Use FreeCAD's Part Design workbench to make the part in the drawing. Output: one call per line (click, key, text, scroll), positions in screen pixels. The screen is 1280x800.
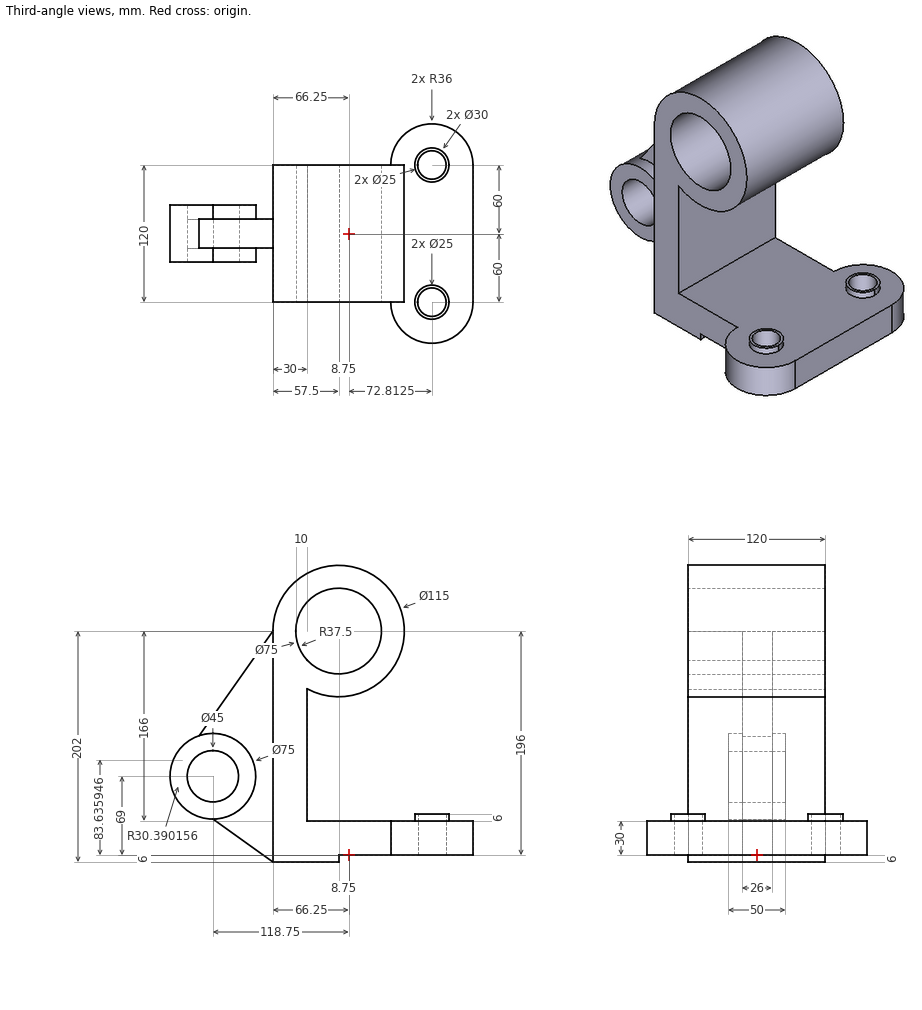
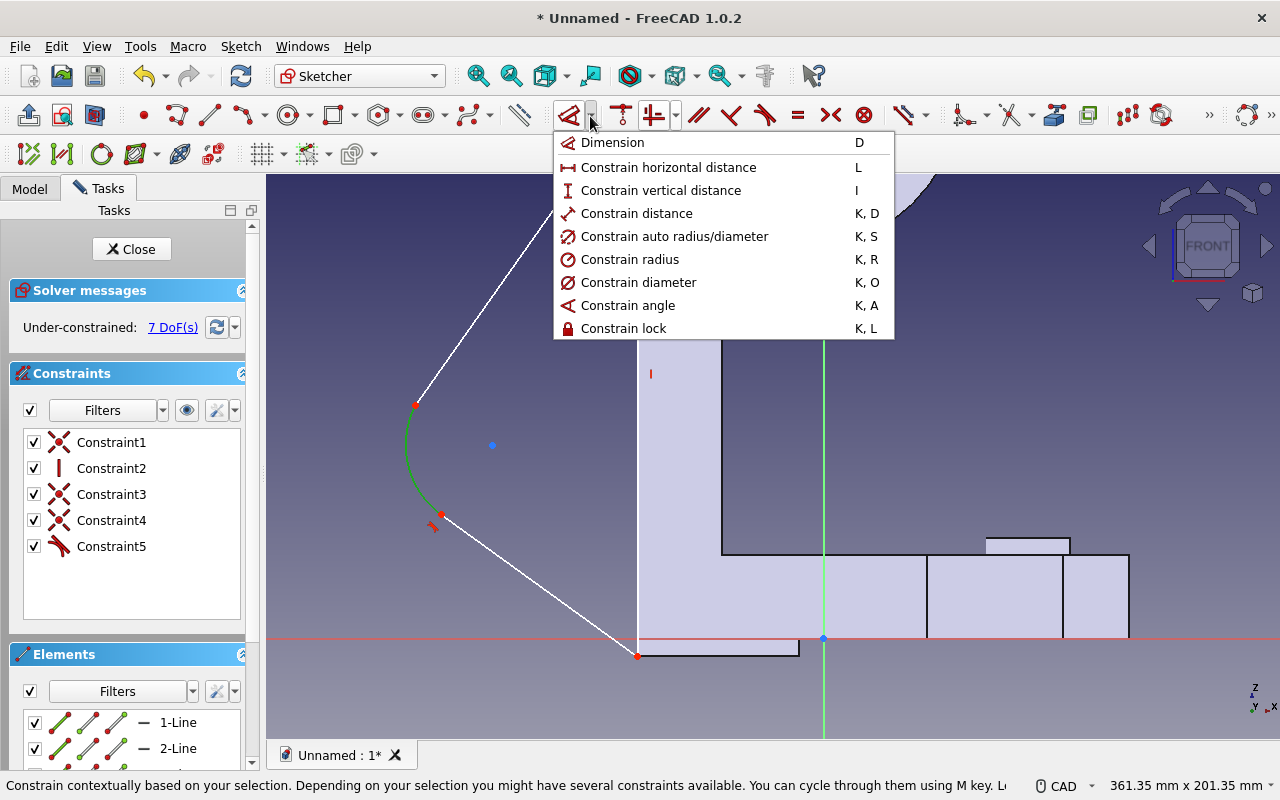
click(724, 260)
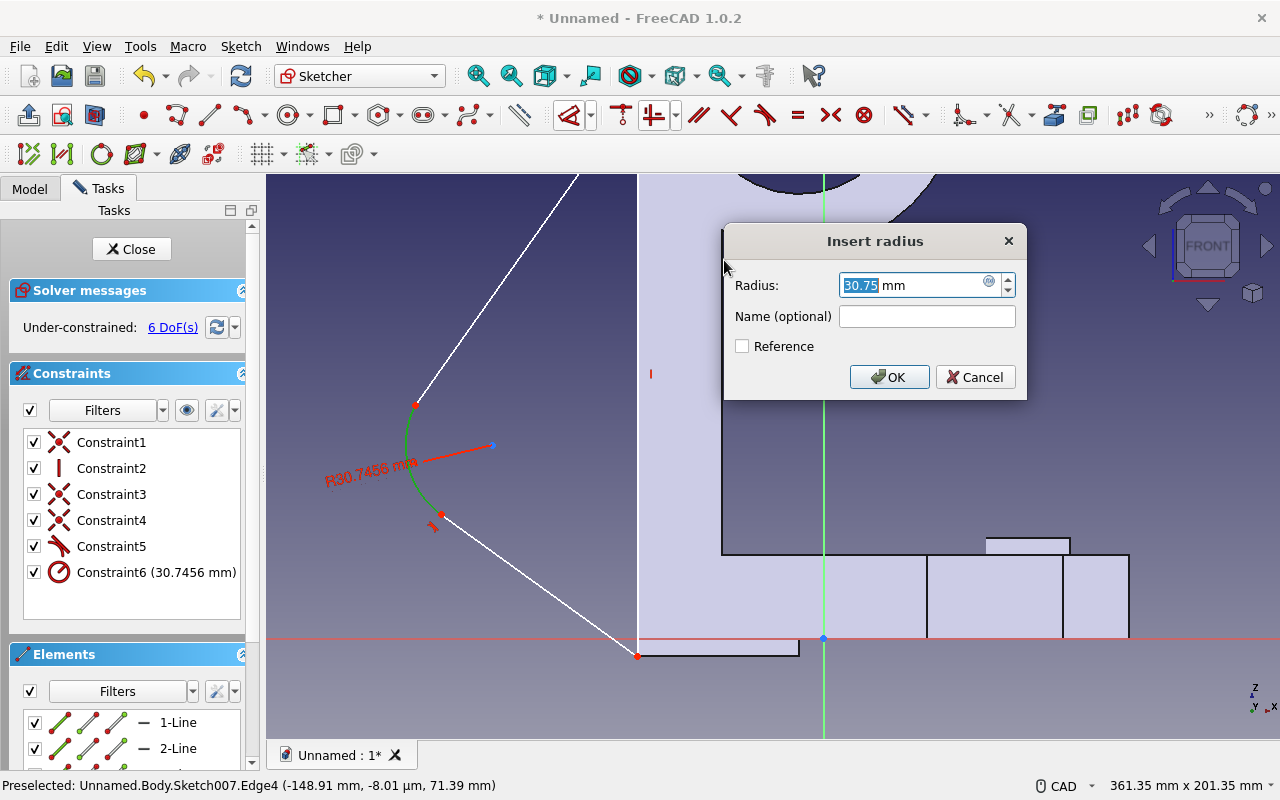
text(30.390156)
key(Return)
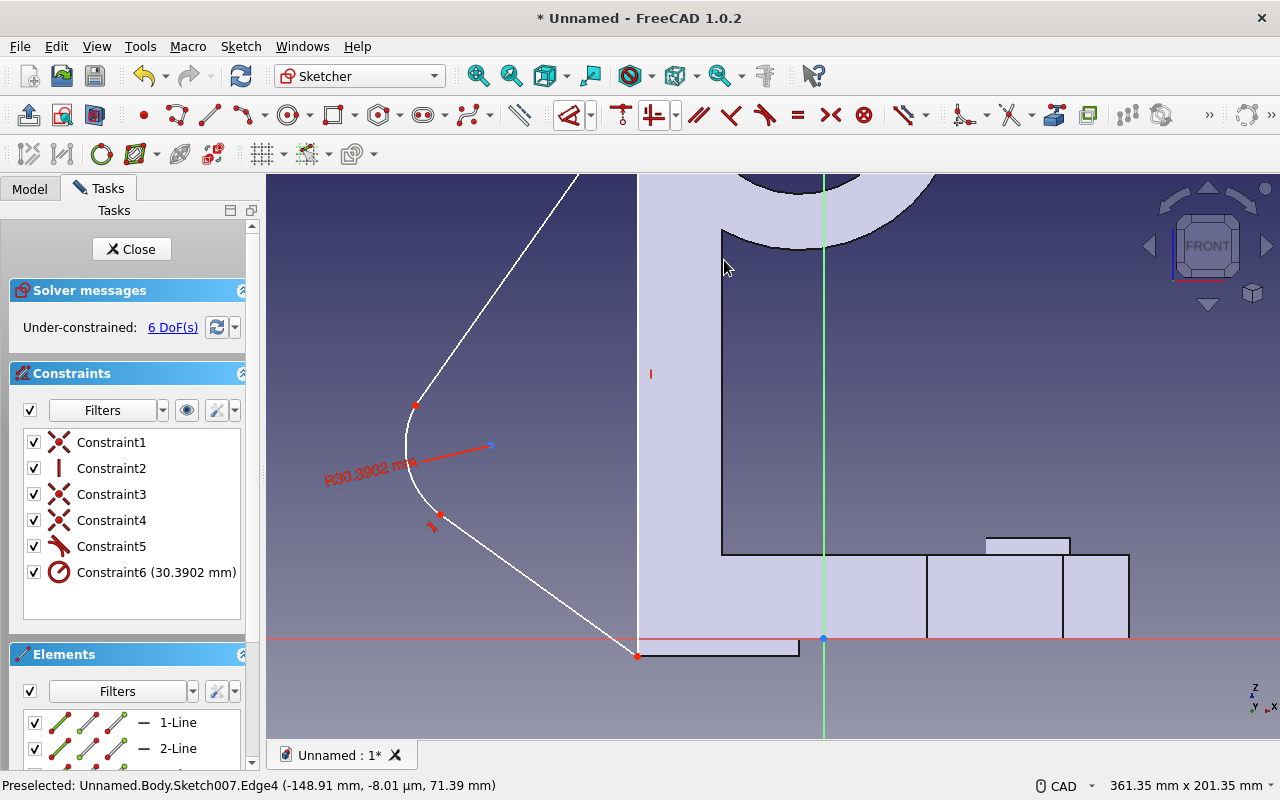
scroll(638, 657, up, 5)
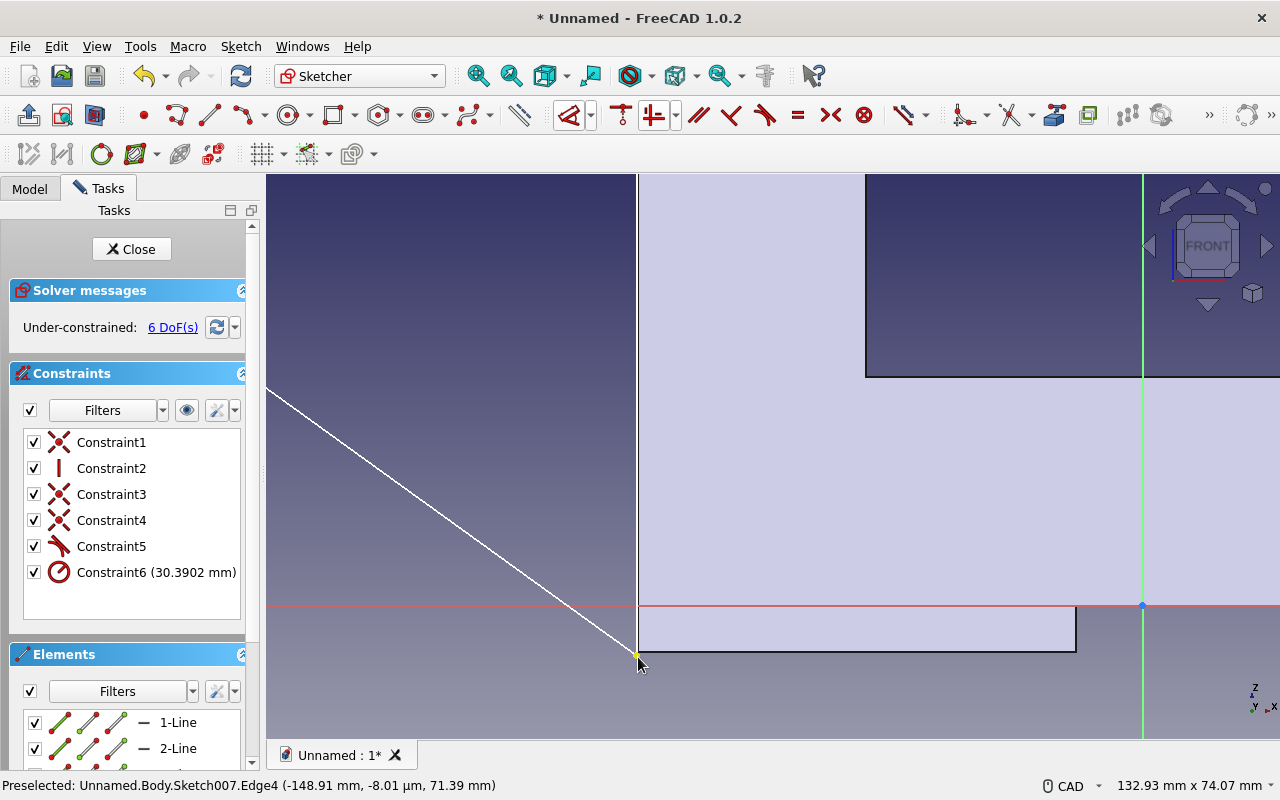
click(637, 656)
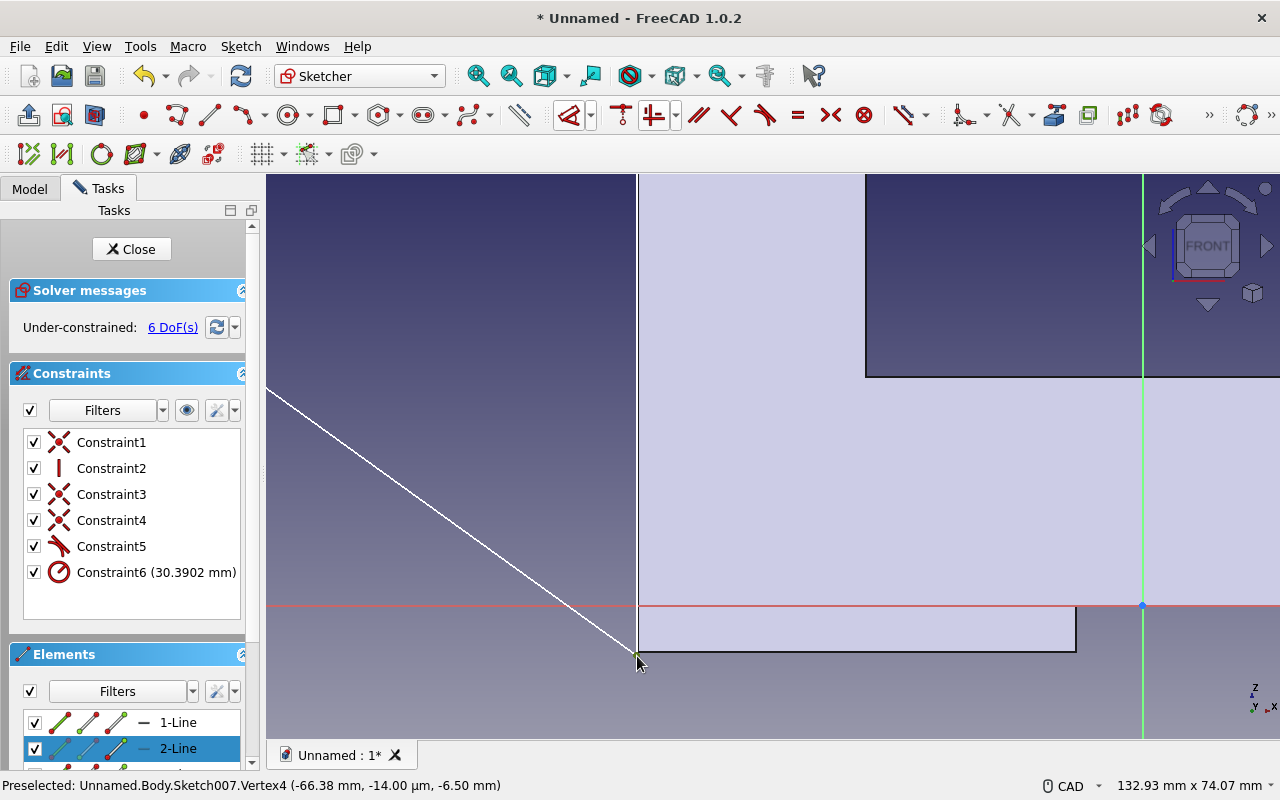
key(i)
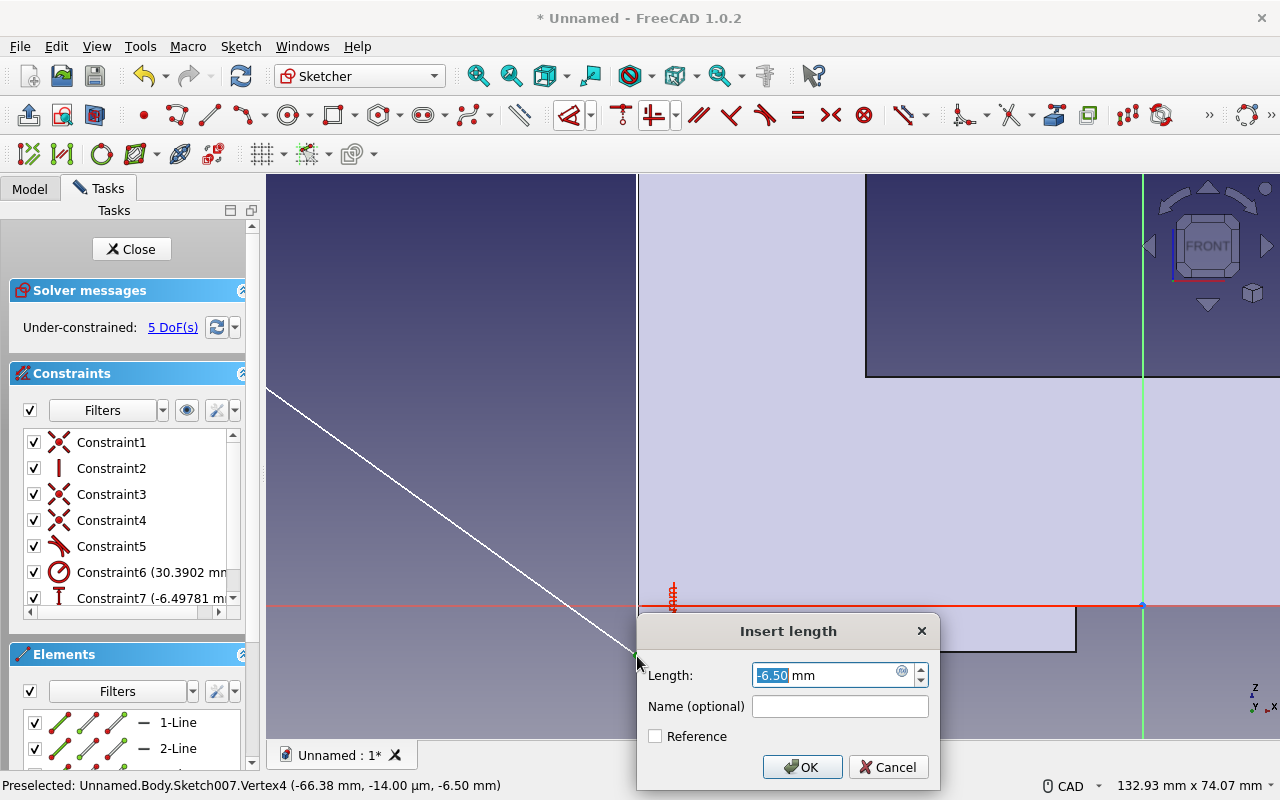
text(-6)
key(Return)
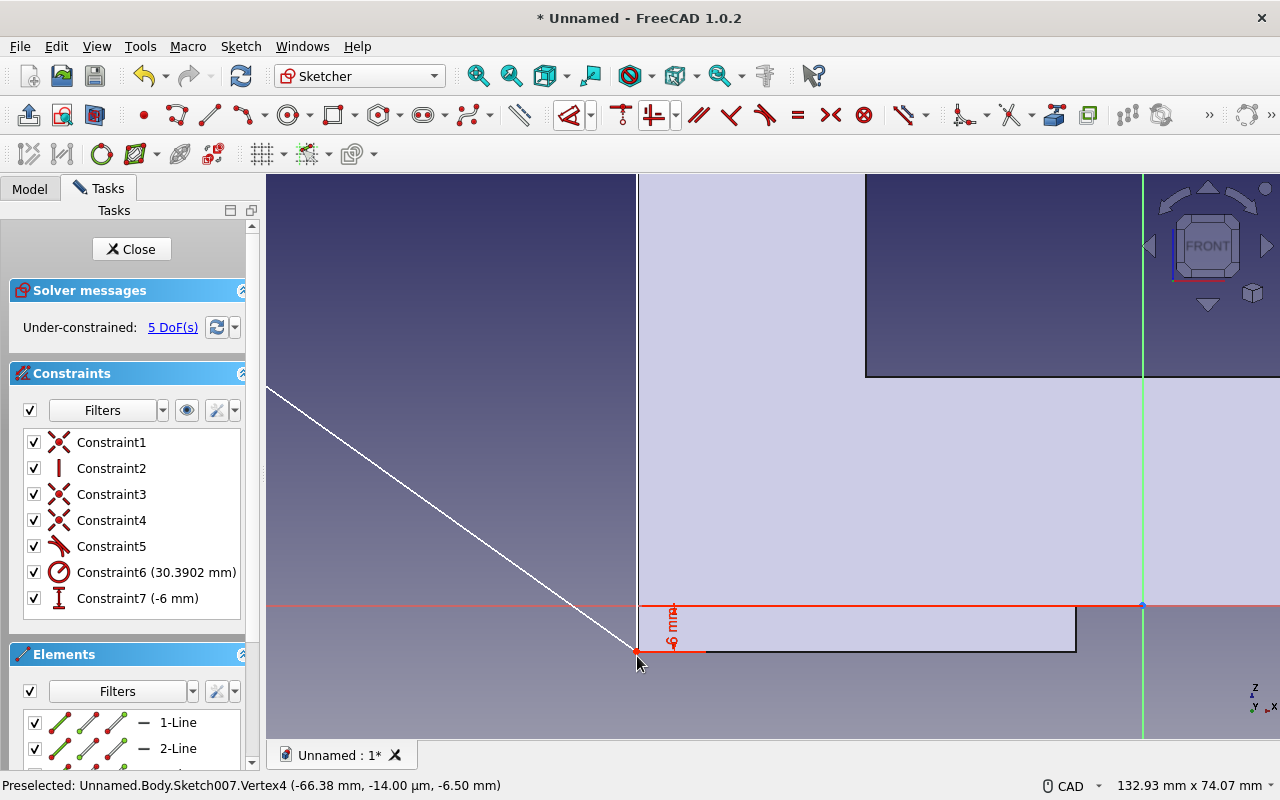
scroll(746, 645, down, 7)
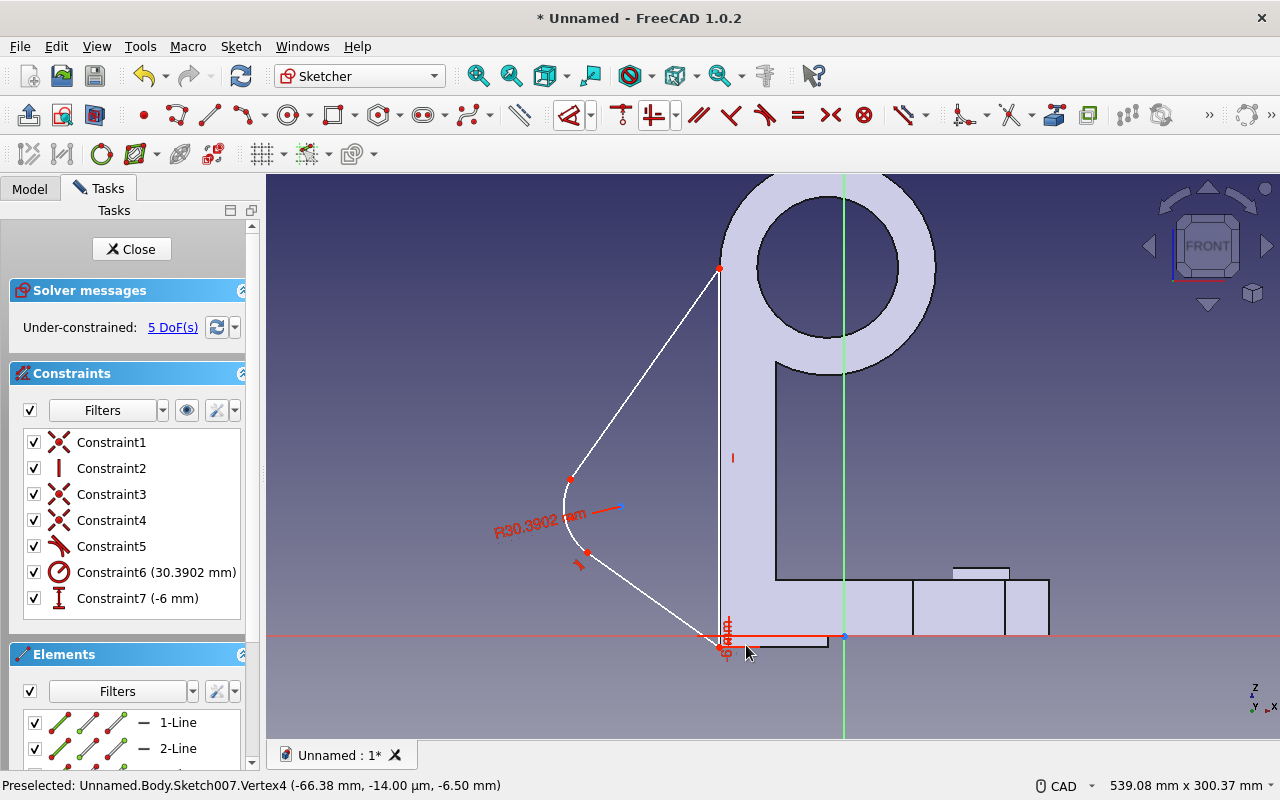
click(719, 572)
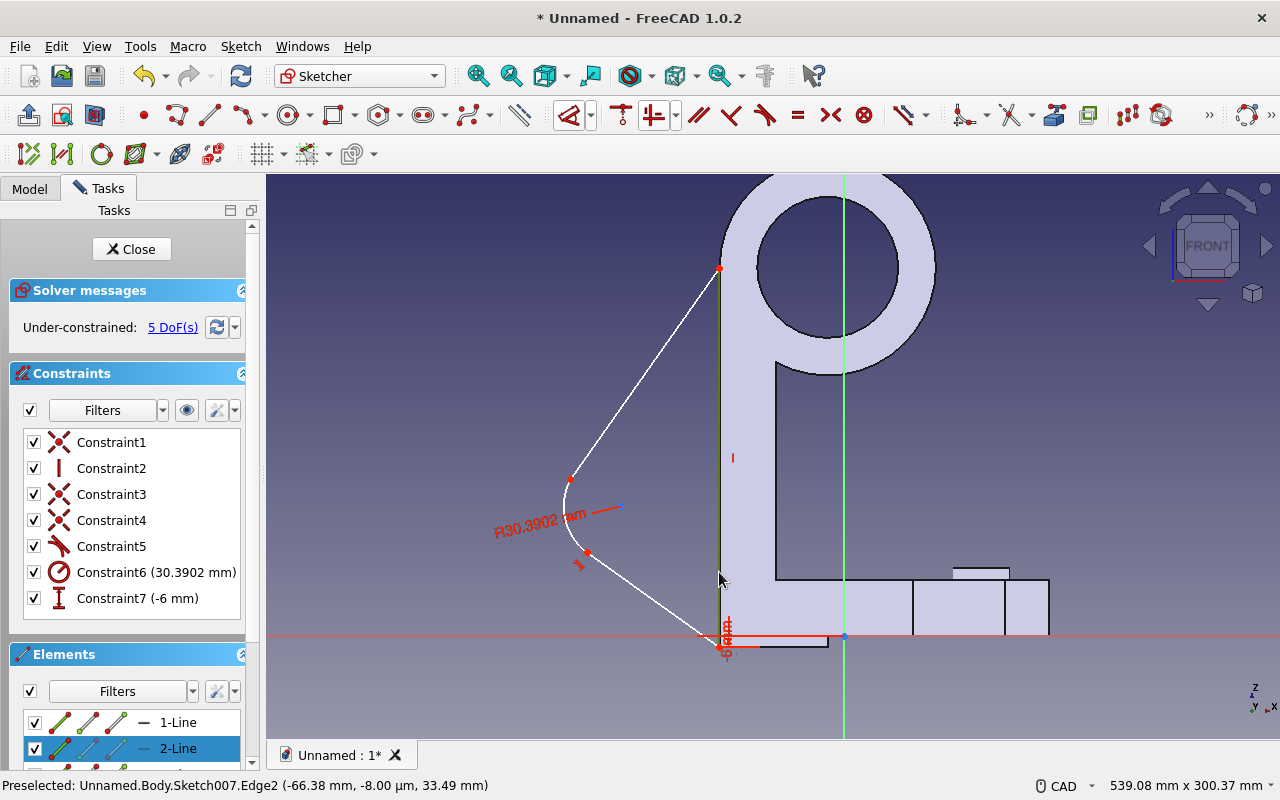
key(i)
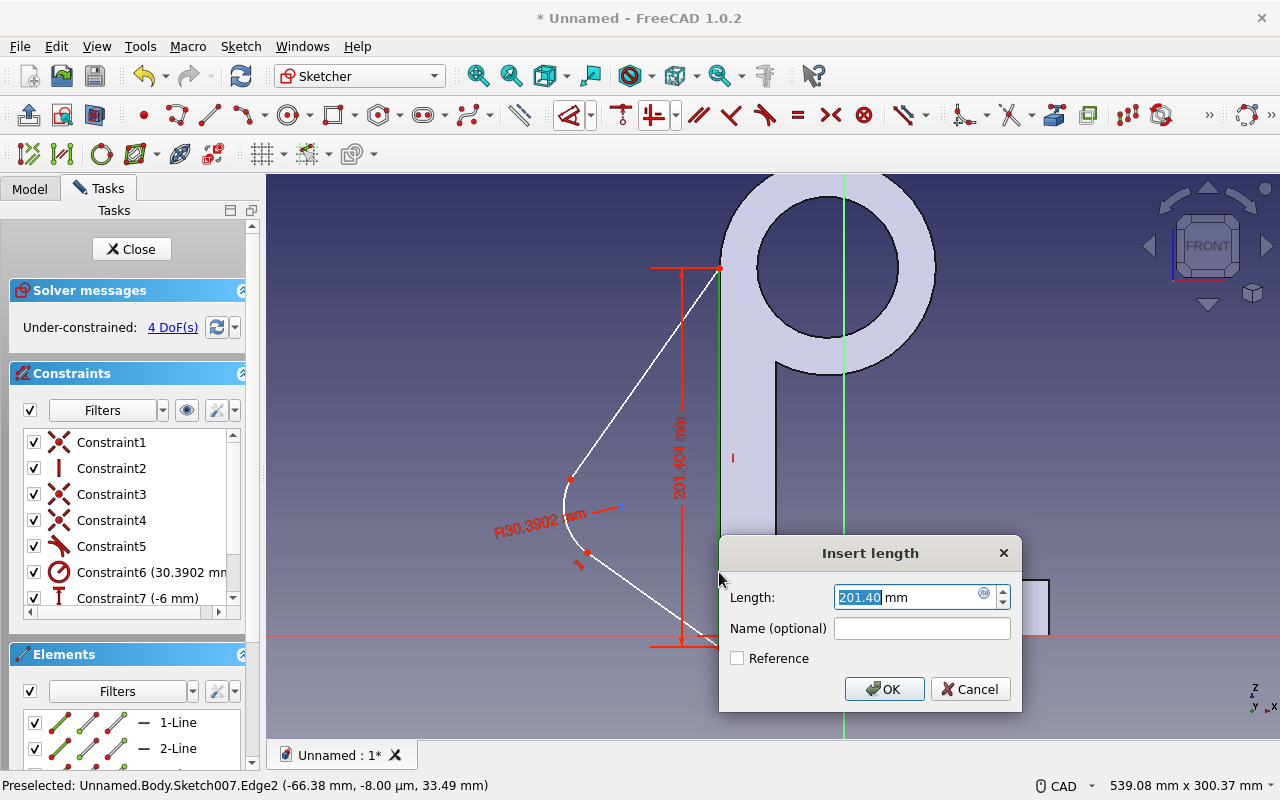
text(202)
key(Return)